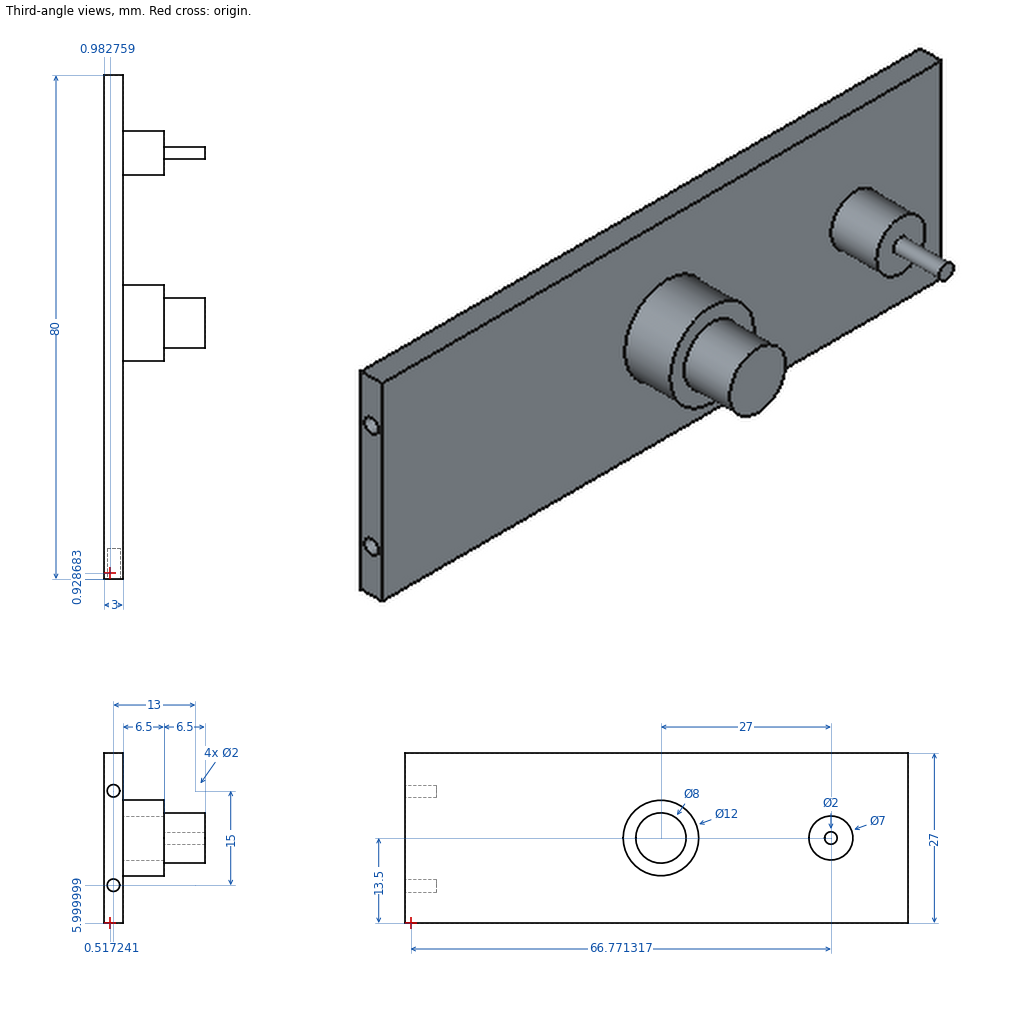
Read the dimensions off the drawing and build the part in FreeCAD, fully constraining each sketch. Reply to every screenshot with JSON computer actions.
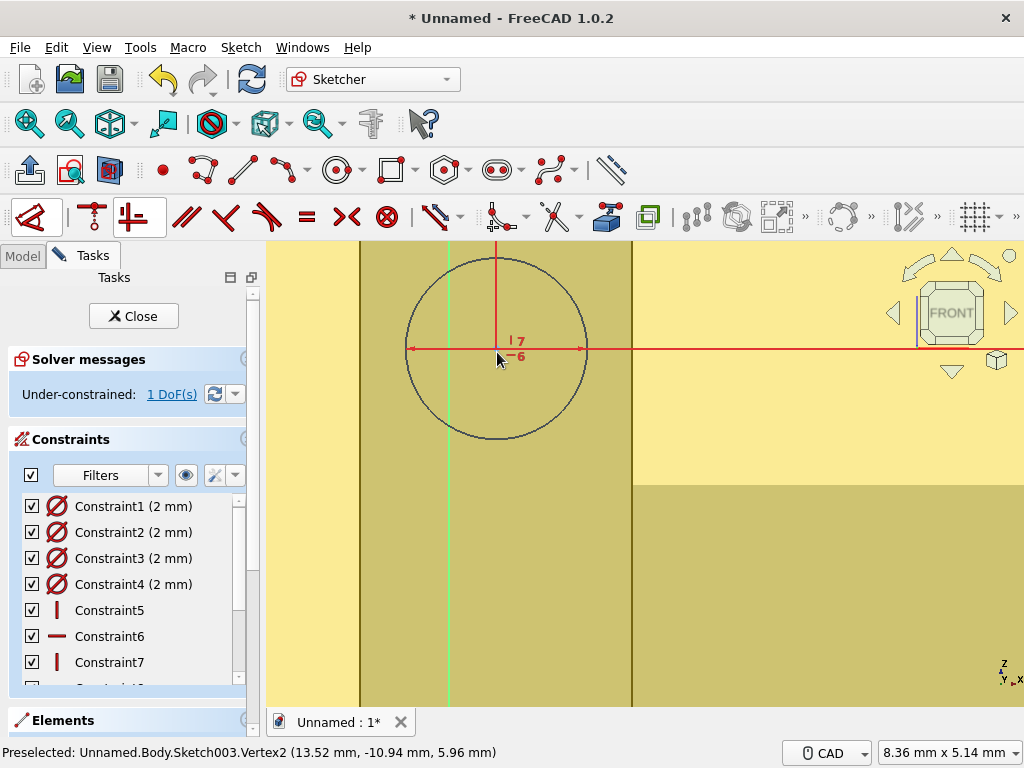
{"action": "left_click", "coordinate": [496, 349]}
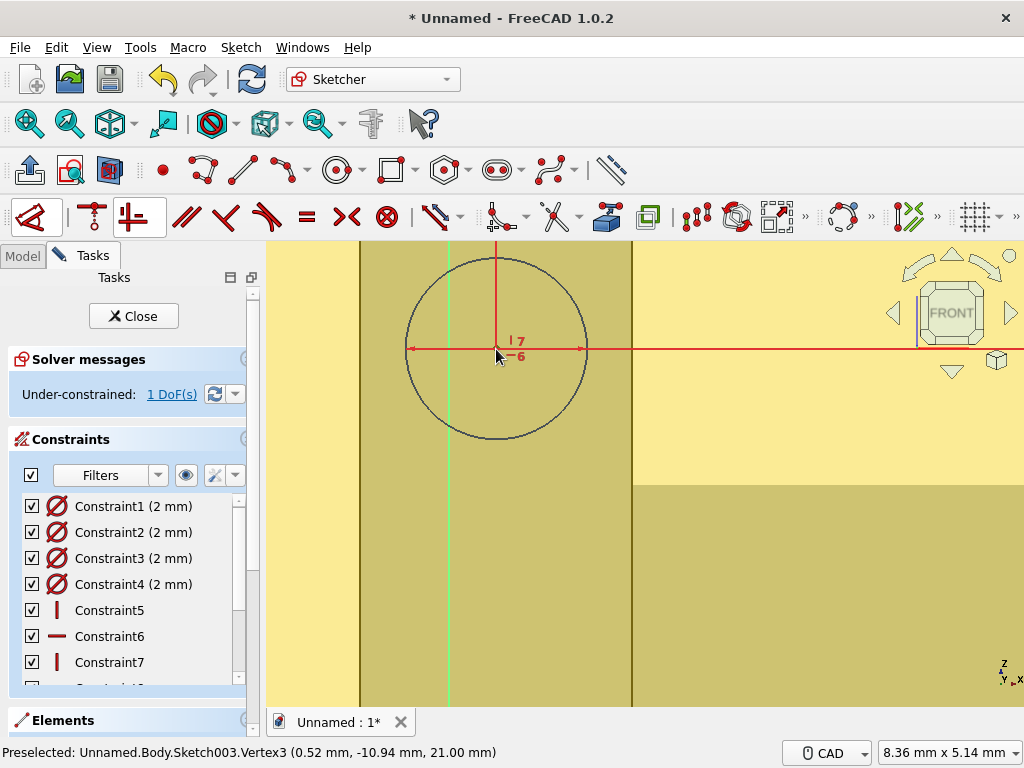
{"action": "left_click", "coordinate": [56, 218]}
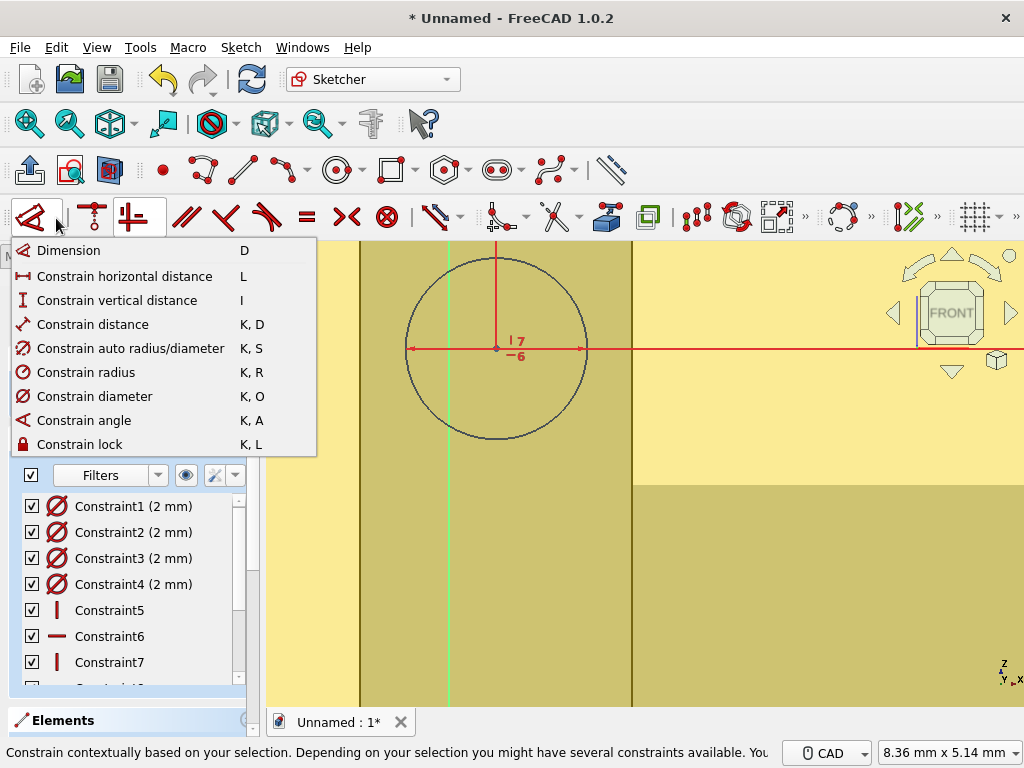
{"action": "left_click", "coordinate": [164, 276]}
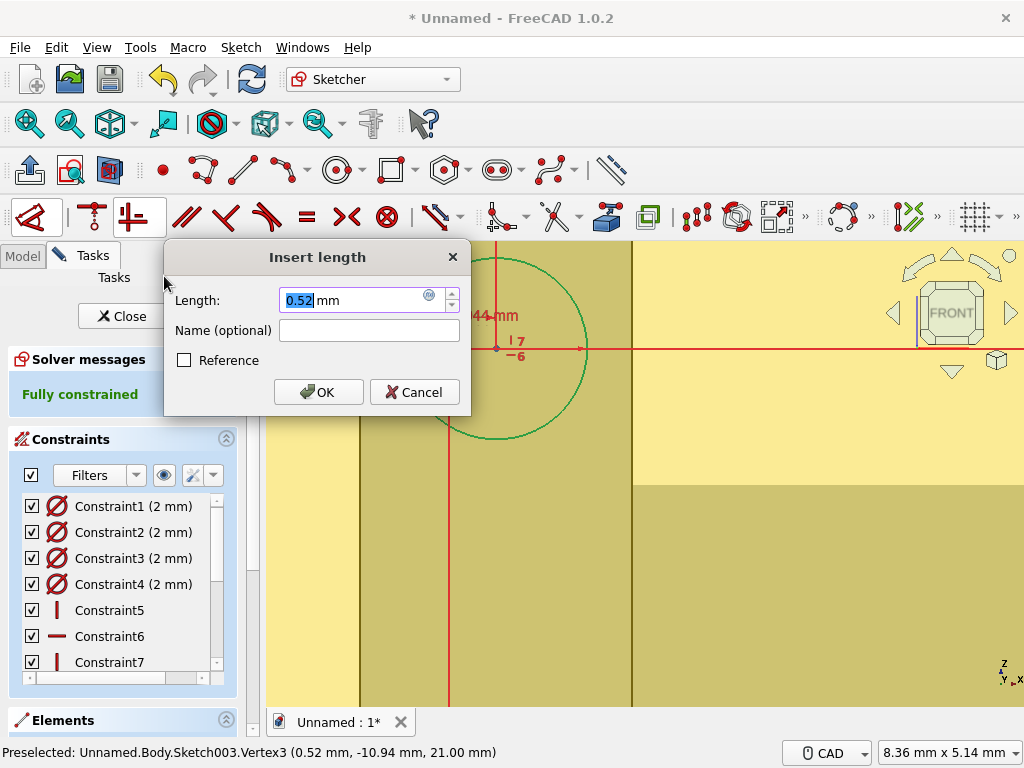
{"action": "type", "text": "0.517241"}
{"action": "key", "text": "Return"}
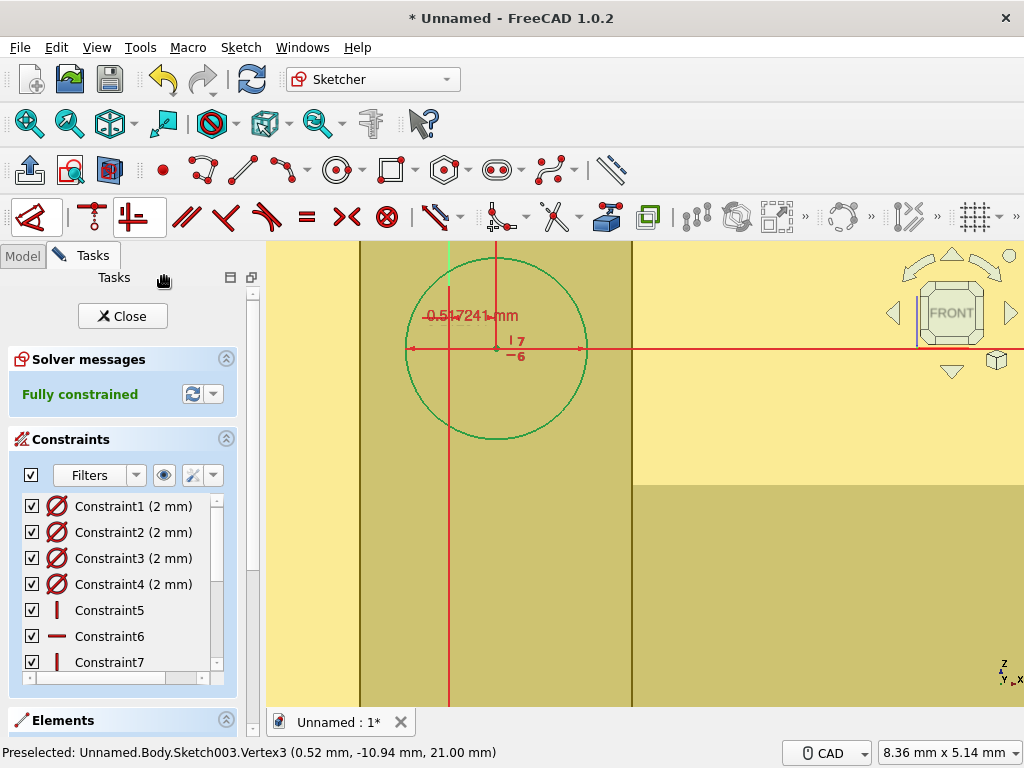
{"action": "left_click", "coordinate": [123, 316]}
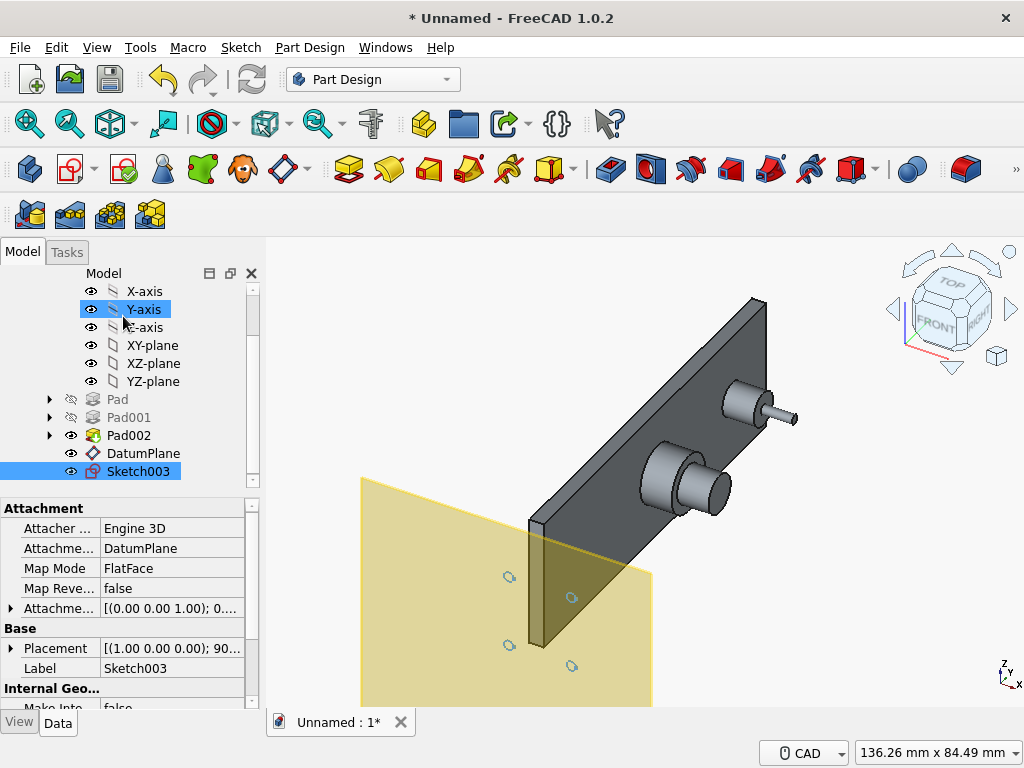
{"action": "left_click", "coordinate": [612, 170]}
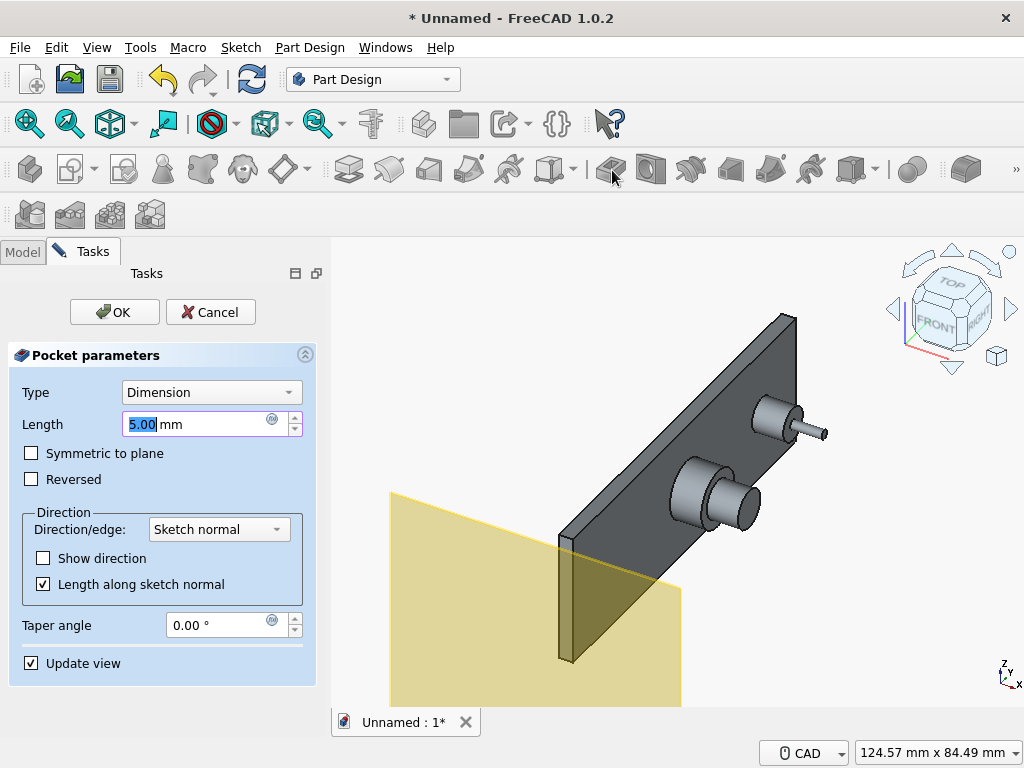
{"action": "type", "text": "15"}
{"action": "key", "text": "Tab"}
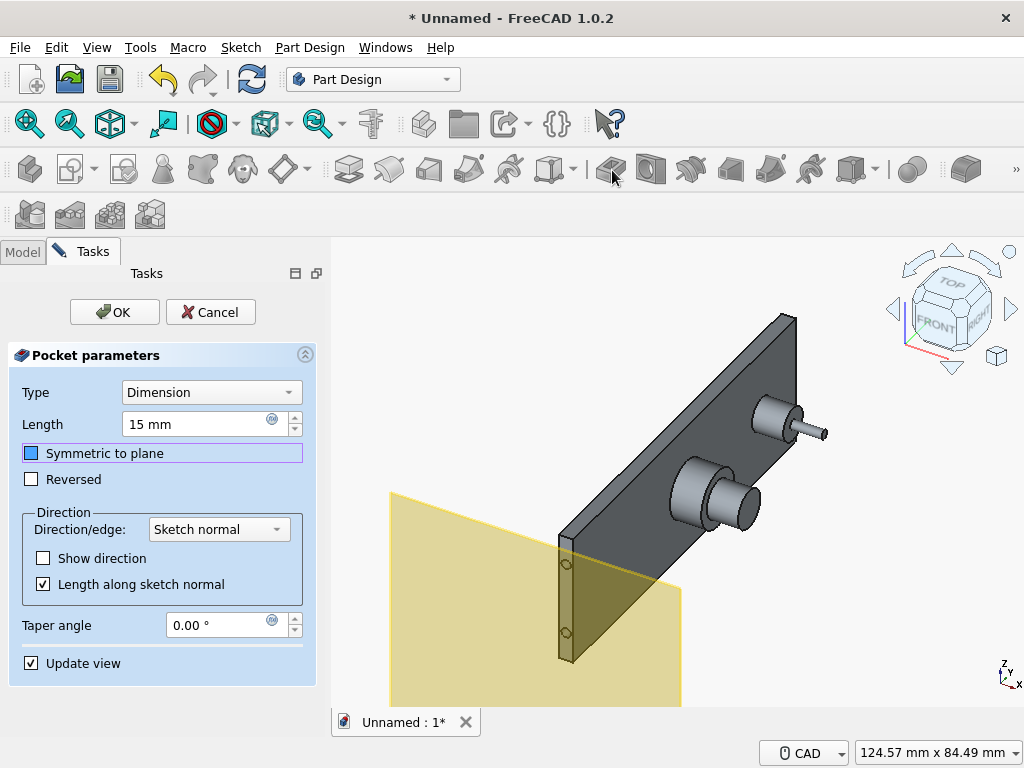
{"action": "left_click", "coordinate": [115, 312]}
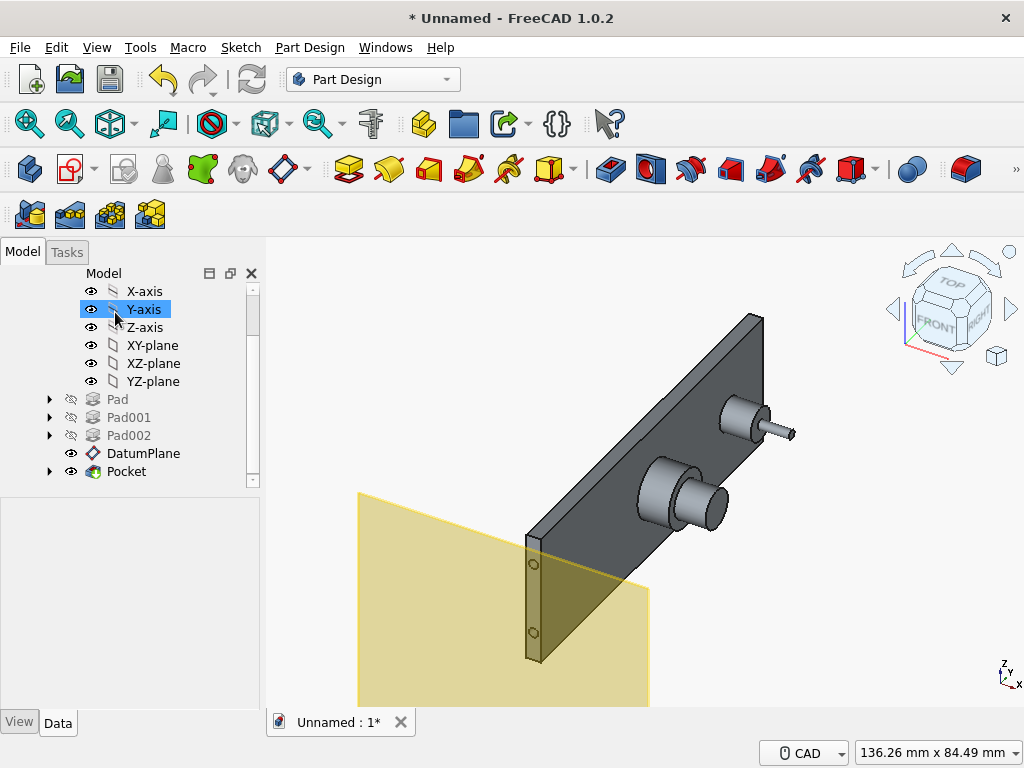
{"action": "left_click", "coordinate": [116, 453]}
{"action": "key", "text": "space"}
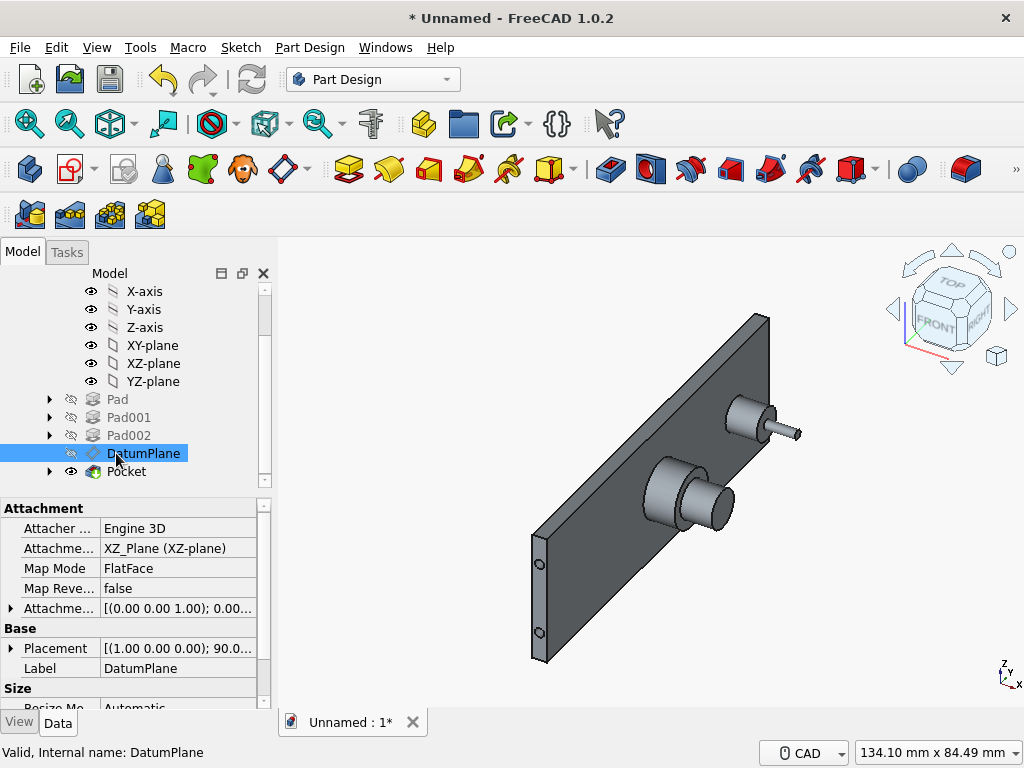
{"action": "key", "text": "0"}